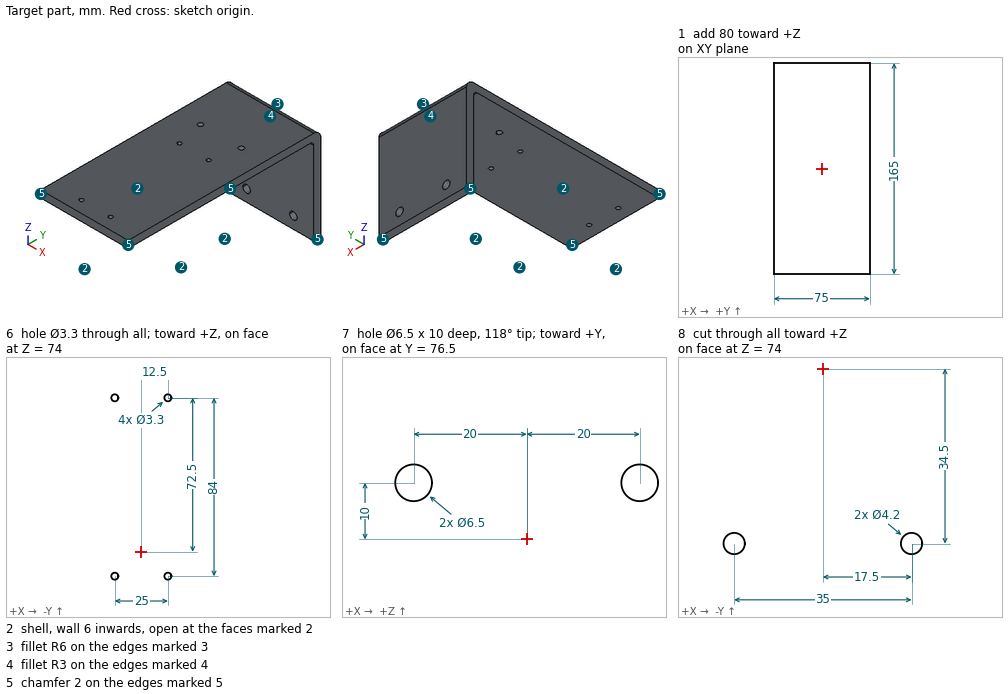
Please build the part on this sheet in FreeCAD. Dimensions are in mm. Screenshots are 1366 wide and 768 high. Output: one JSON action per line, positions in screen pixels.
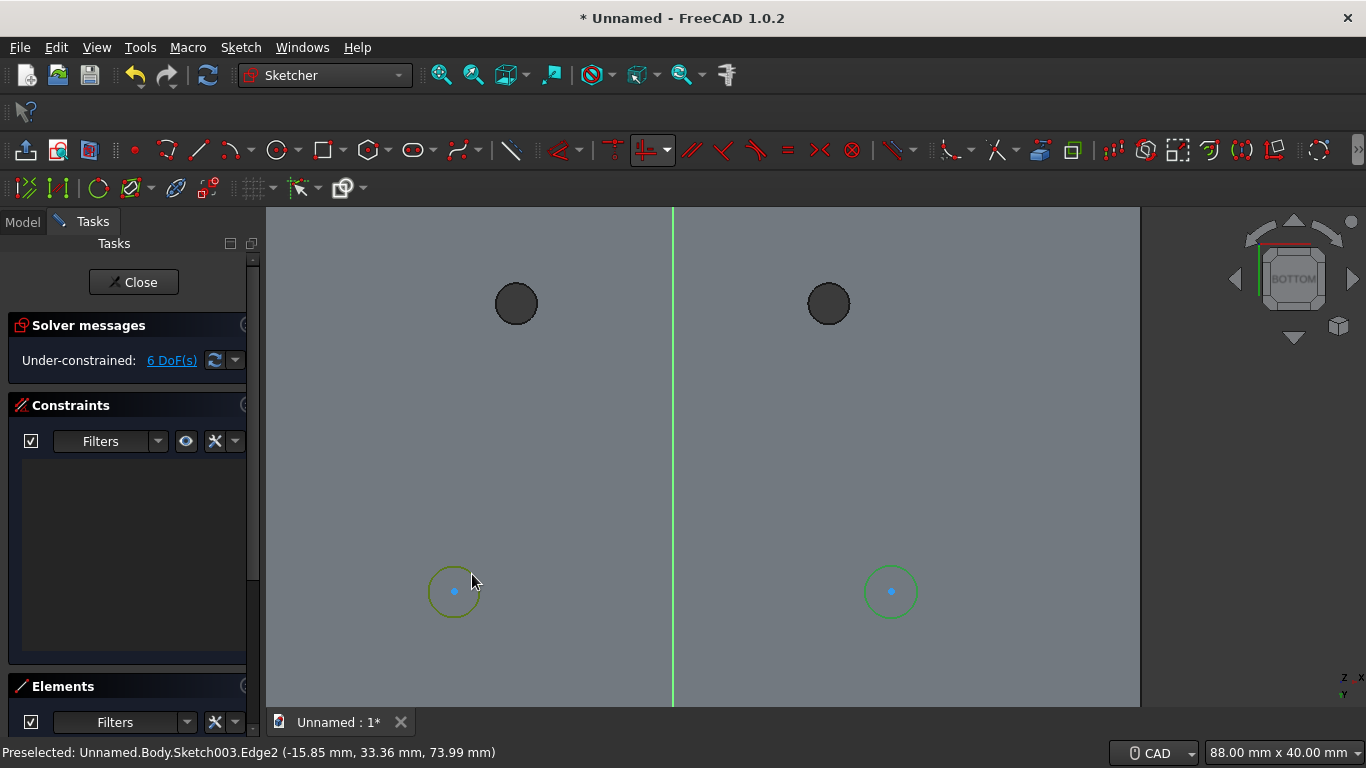
{"action": "left_click", "coordinate": [788, 150]}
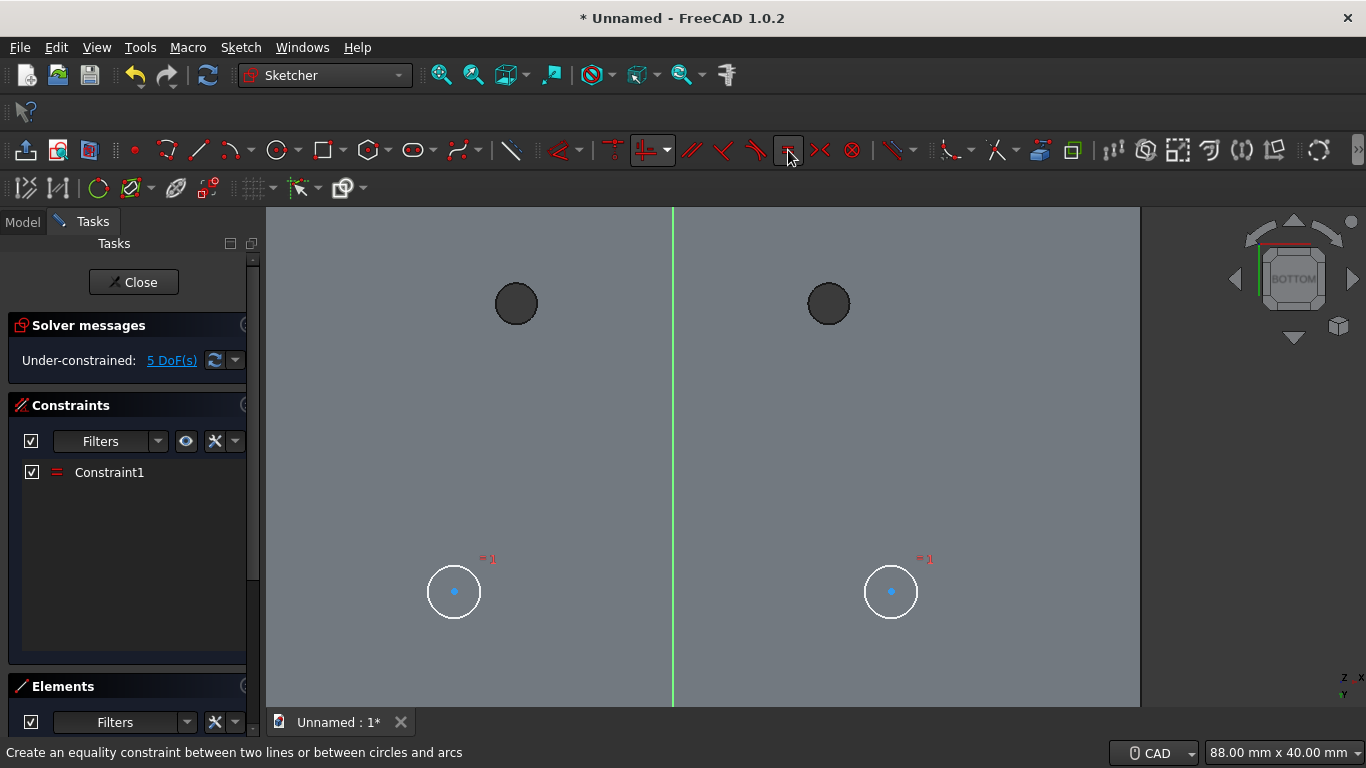
{"action": "left_click", "coordinate": [891, 592]}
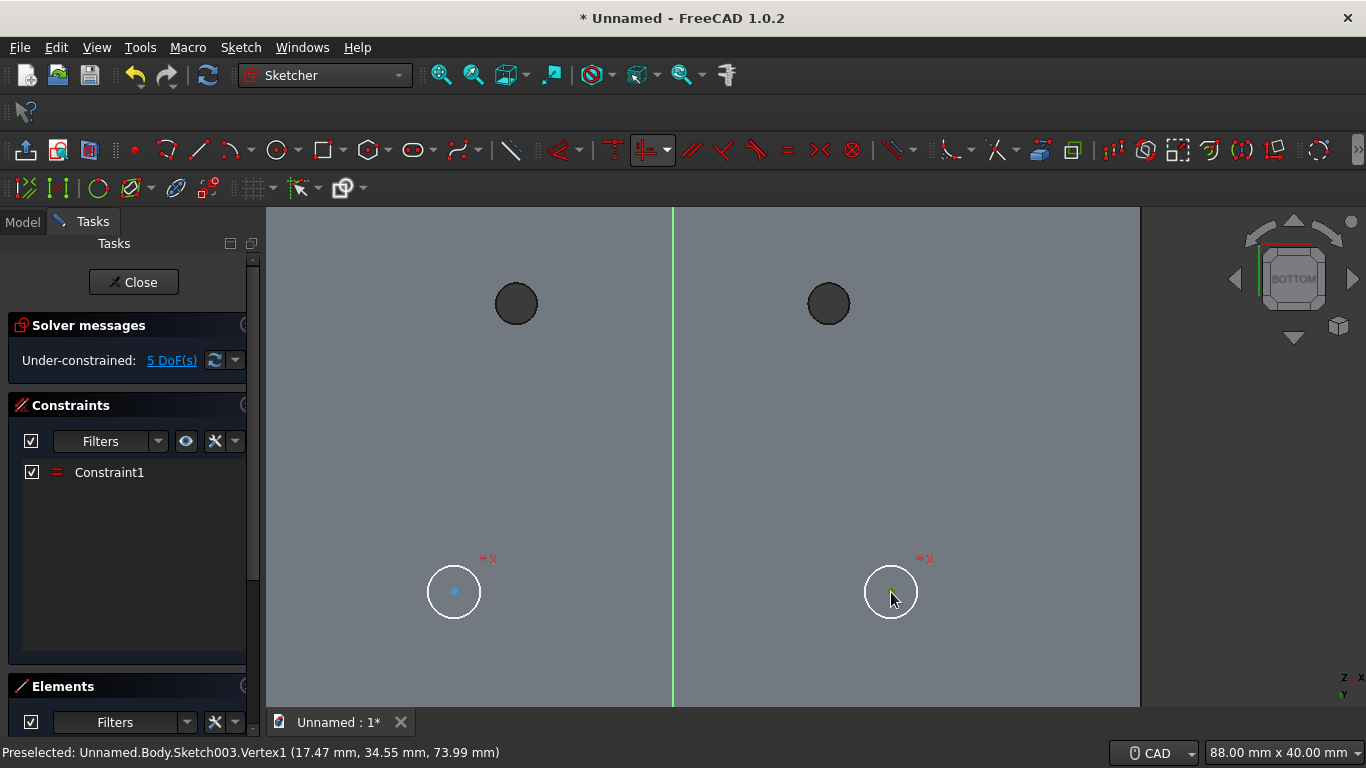
{"action": "left_click", "coordinate": [454, 592]}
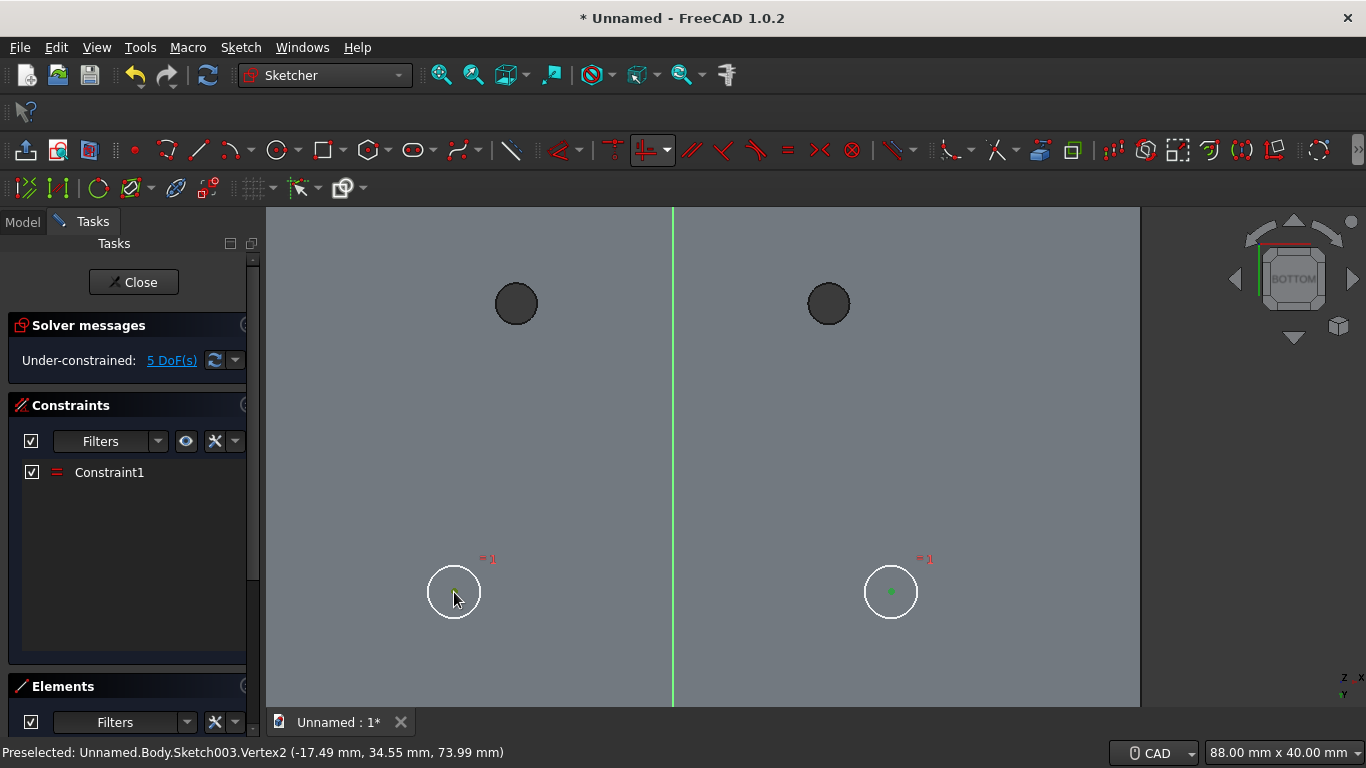
{"action": "left_click", "coordinate": [670, 150]}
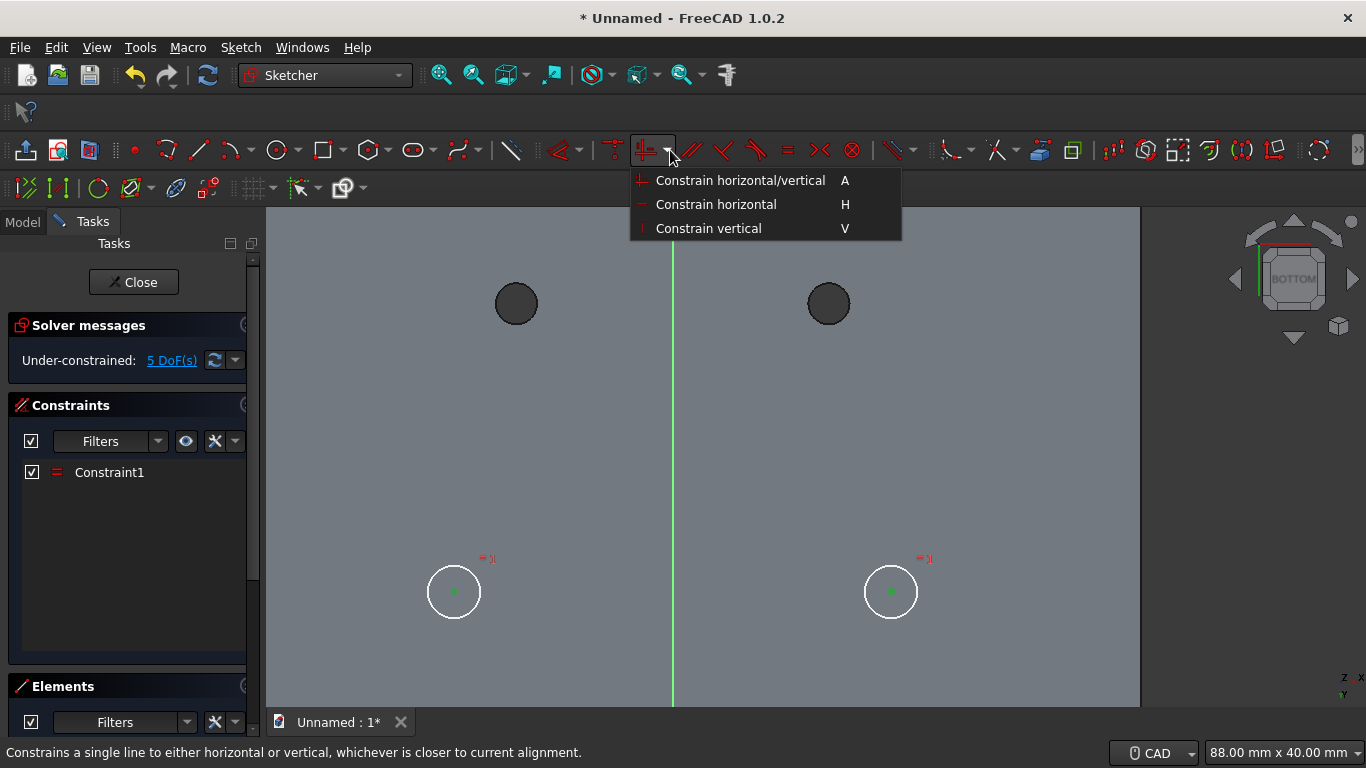
{"action": "left_click", "coordinate": [766, 204]}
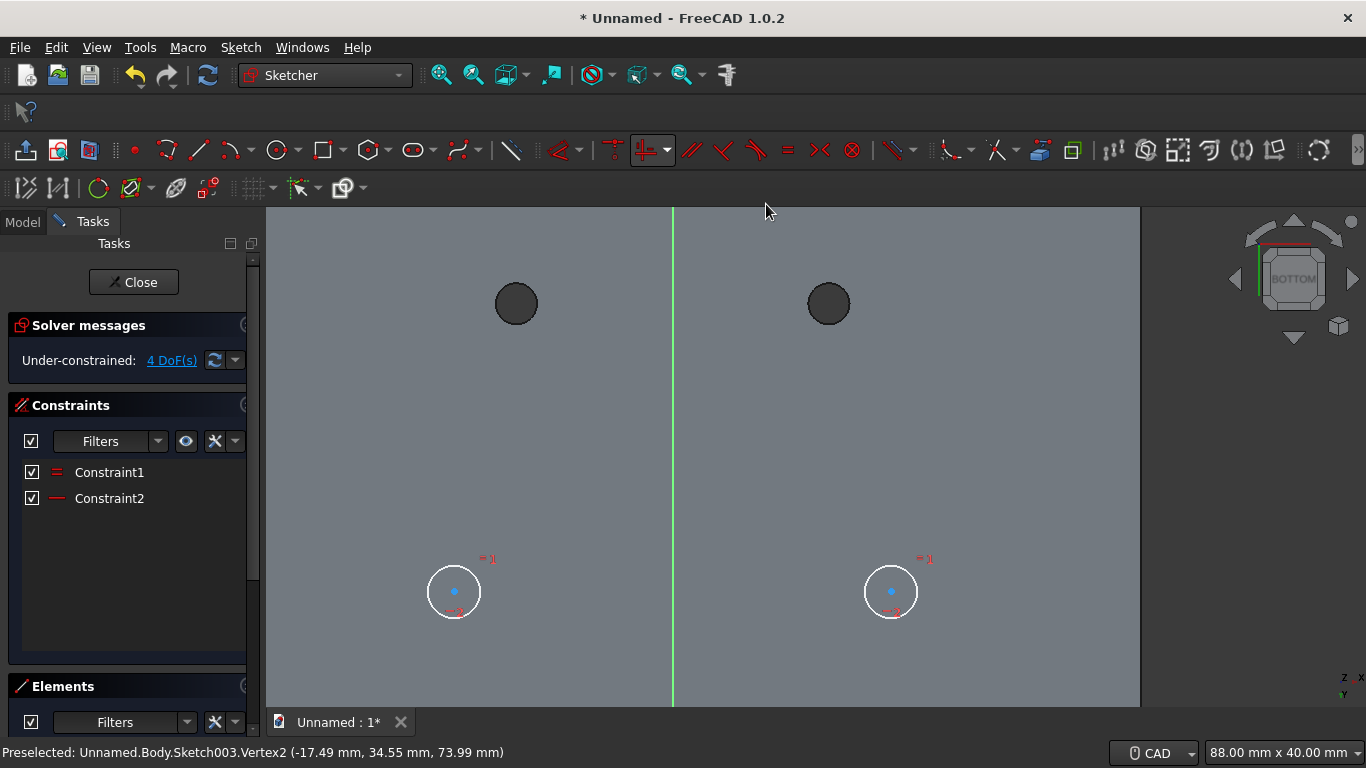
{"action": "left_click", "coordinate": [558, 150]}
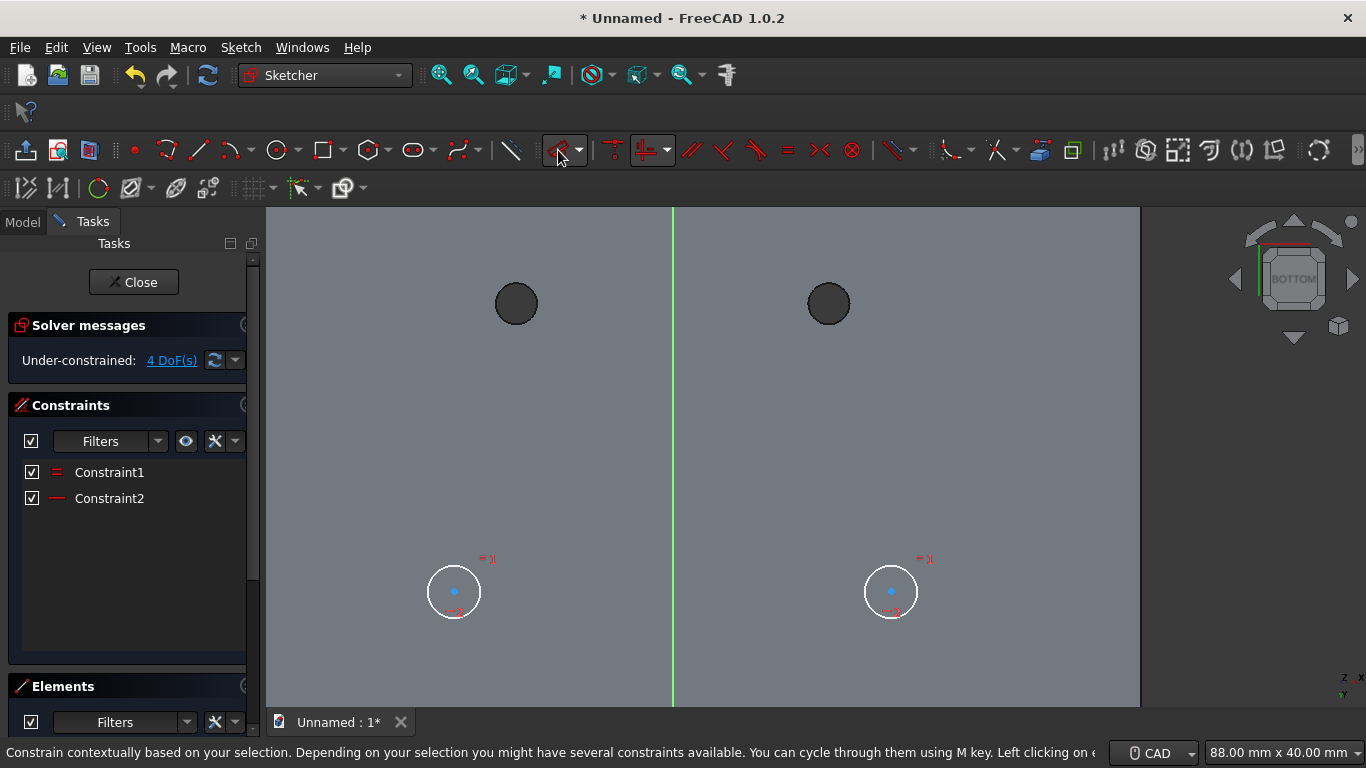
{"action": "left_click", "coordinate": [909, 573]}
{"action": "left_click", "coordinate": [931, 550]}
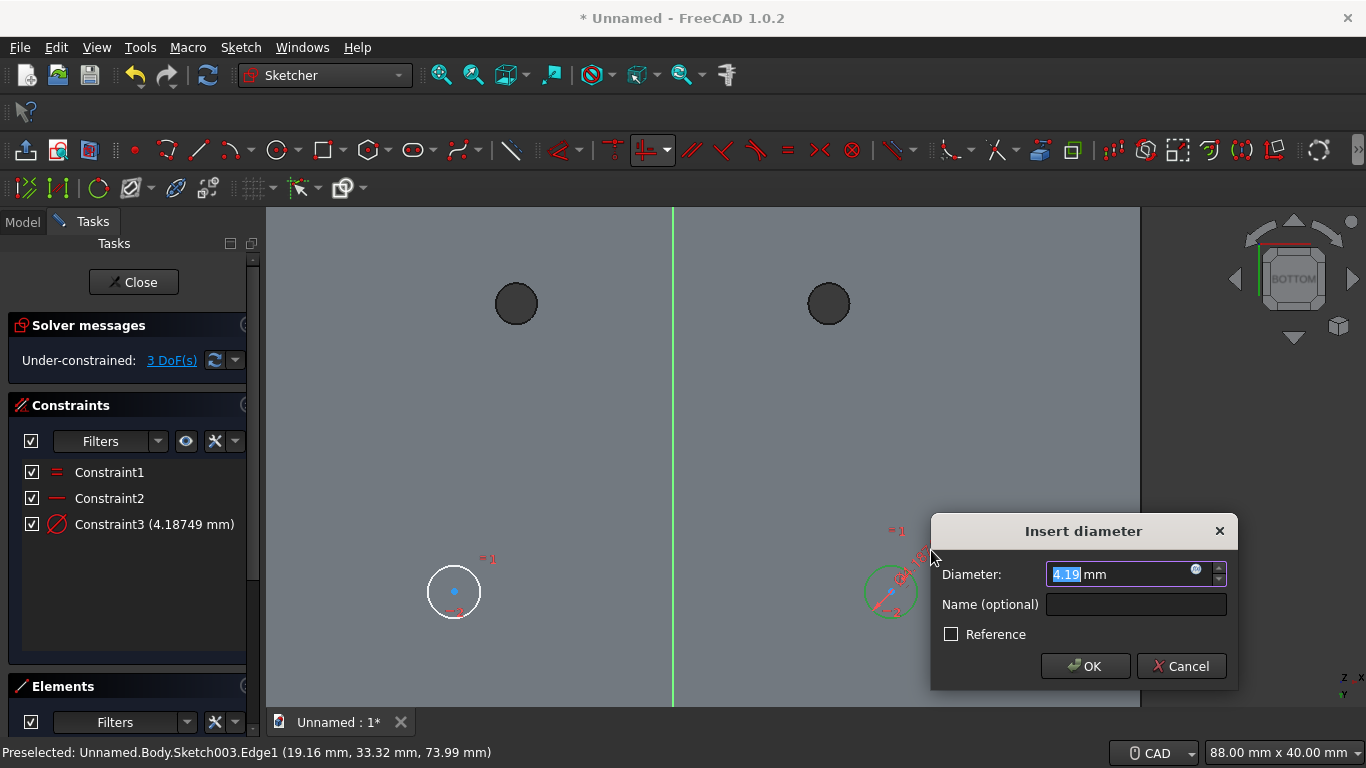
{"action": "type", "text": "4.2"}
{"action": "key", "text": "Return"}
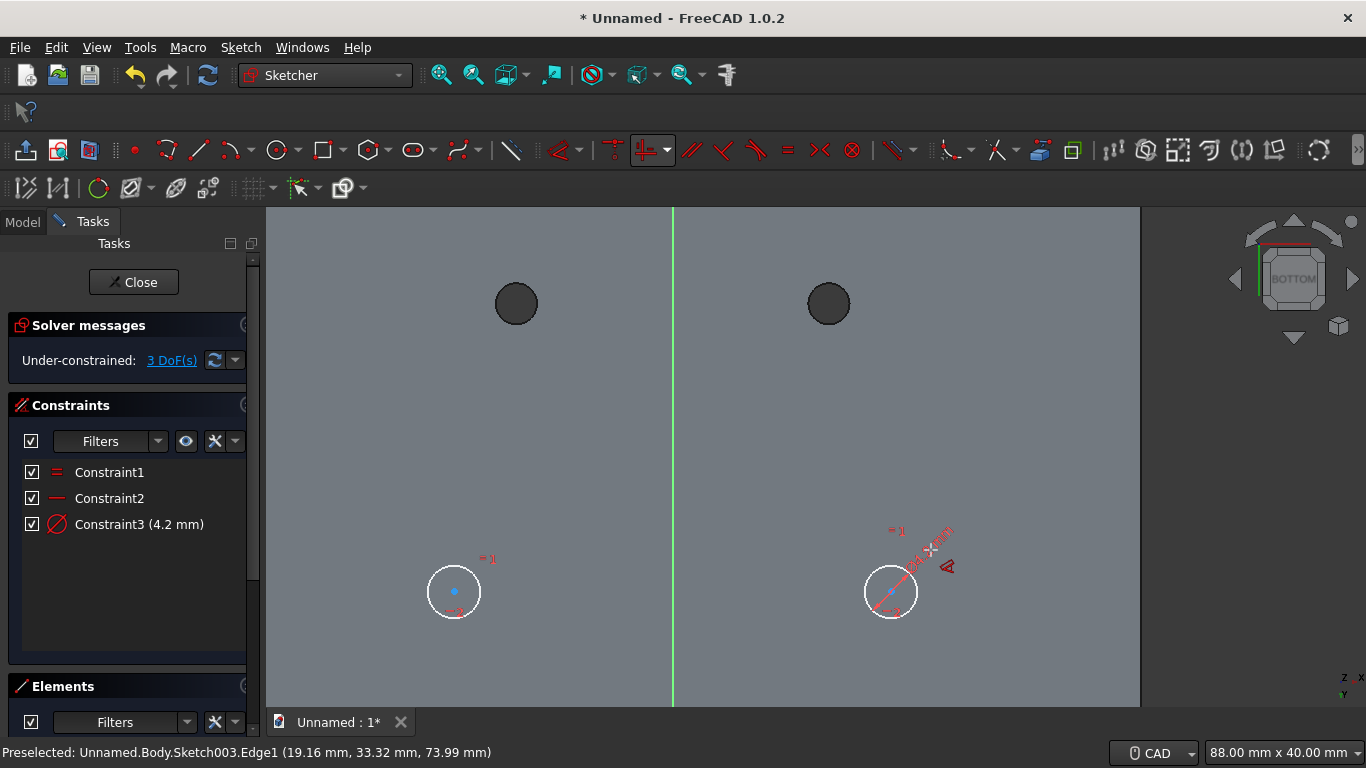
{"action": "left_click", "coordinate": [891, 592]}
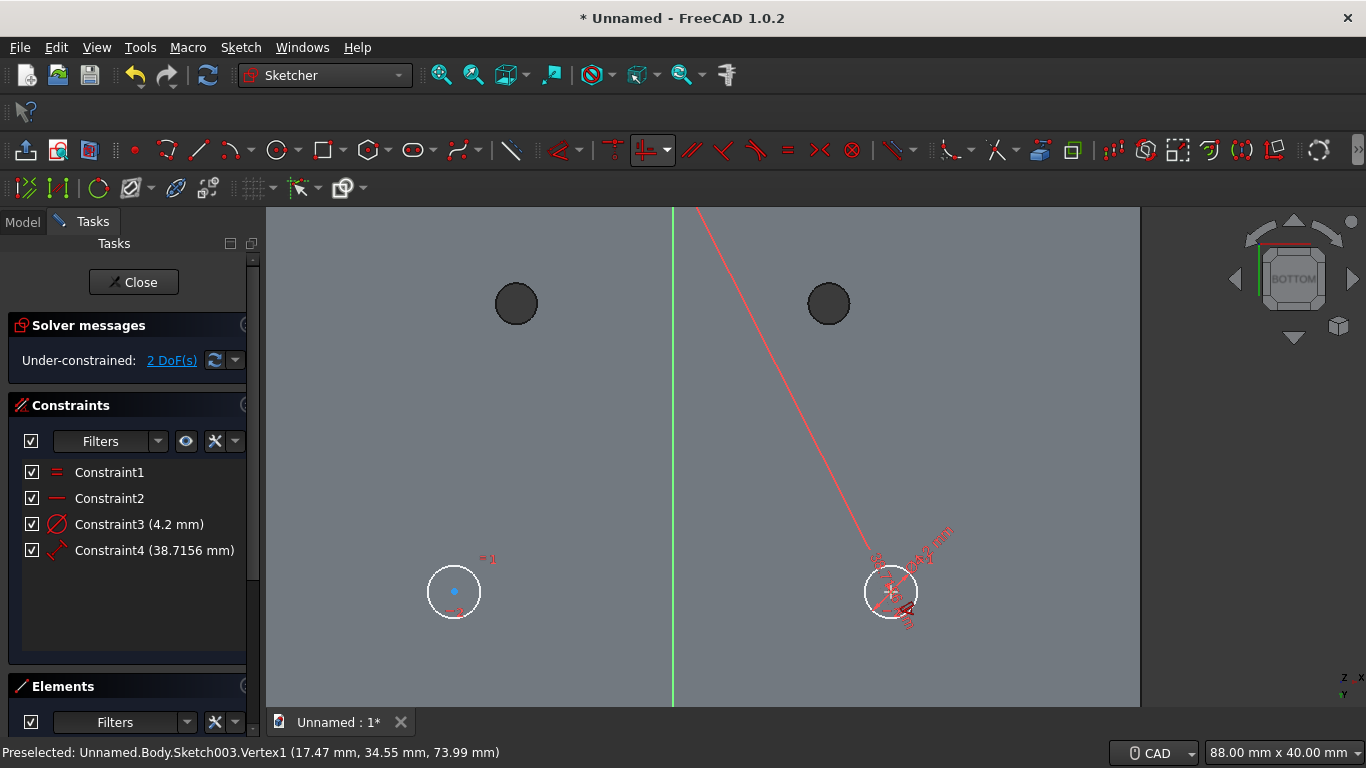
{"action": "left_click", "coordinate": [454, 592]}
{"action": "left_click", "coordinate": [572, 626]}